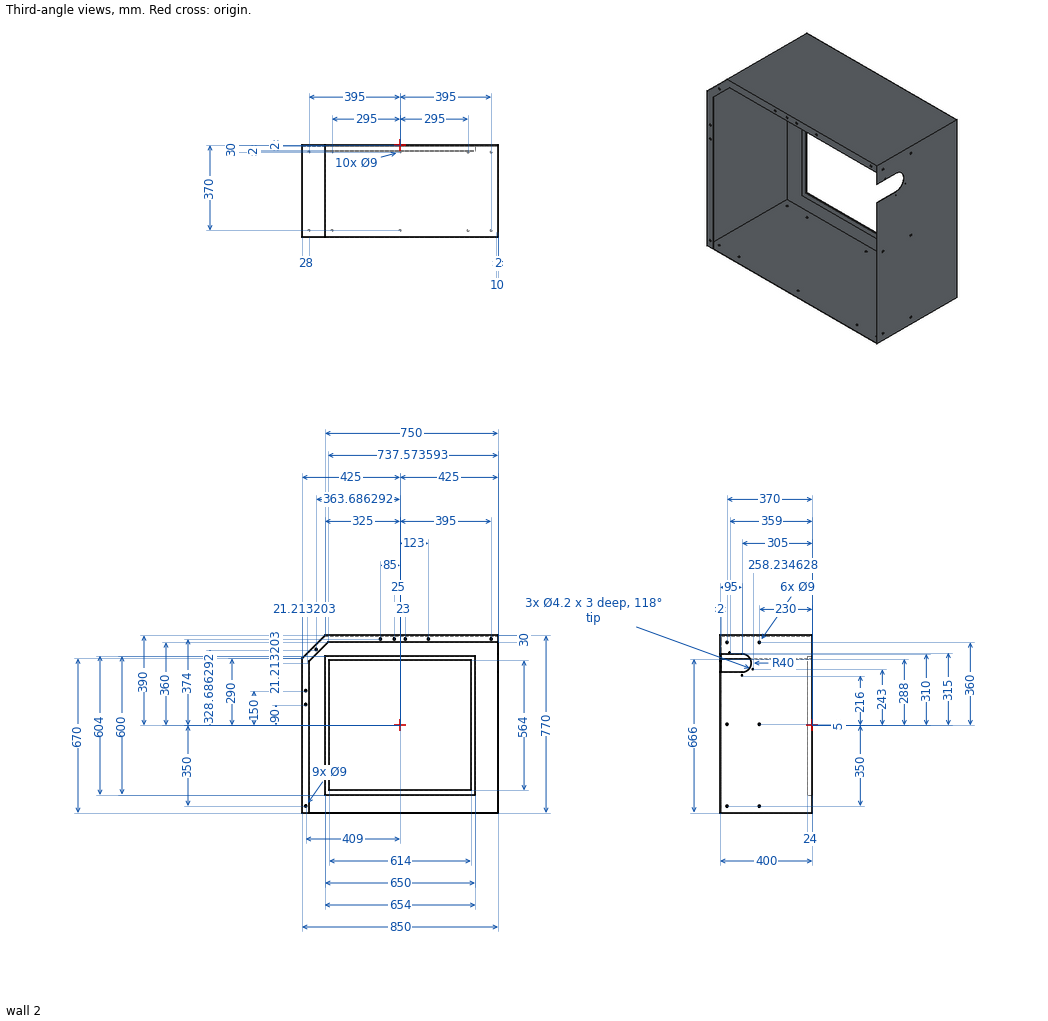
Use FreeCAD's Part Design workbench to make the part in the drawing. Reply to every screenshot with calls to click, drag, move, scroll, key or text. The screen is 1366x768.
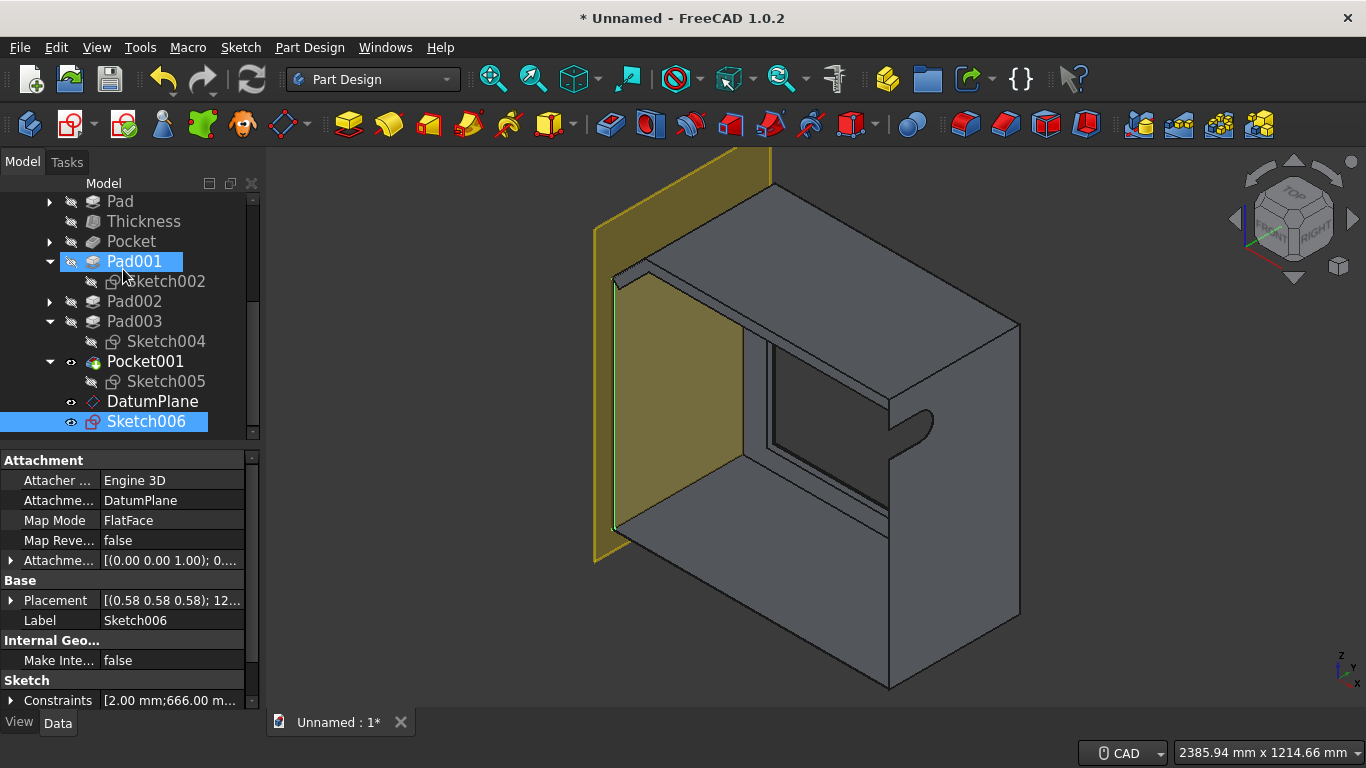
click(350, 124)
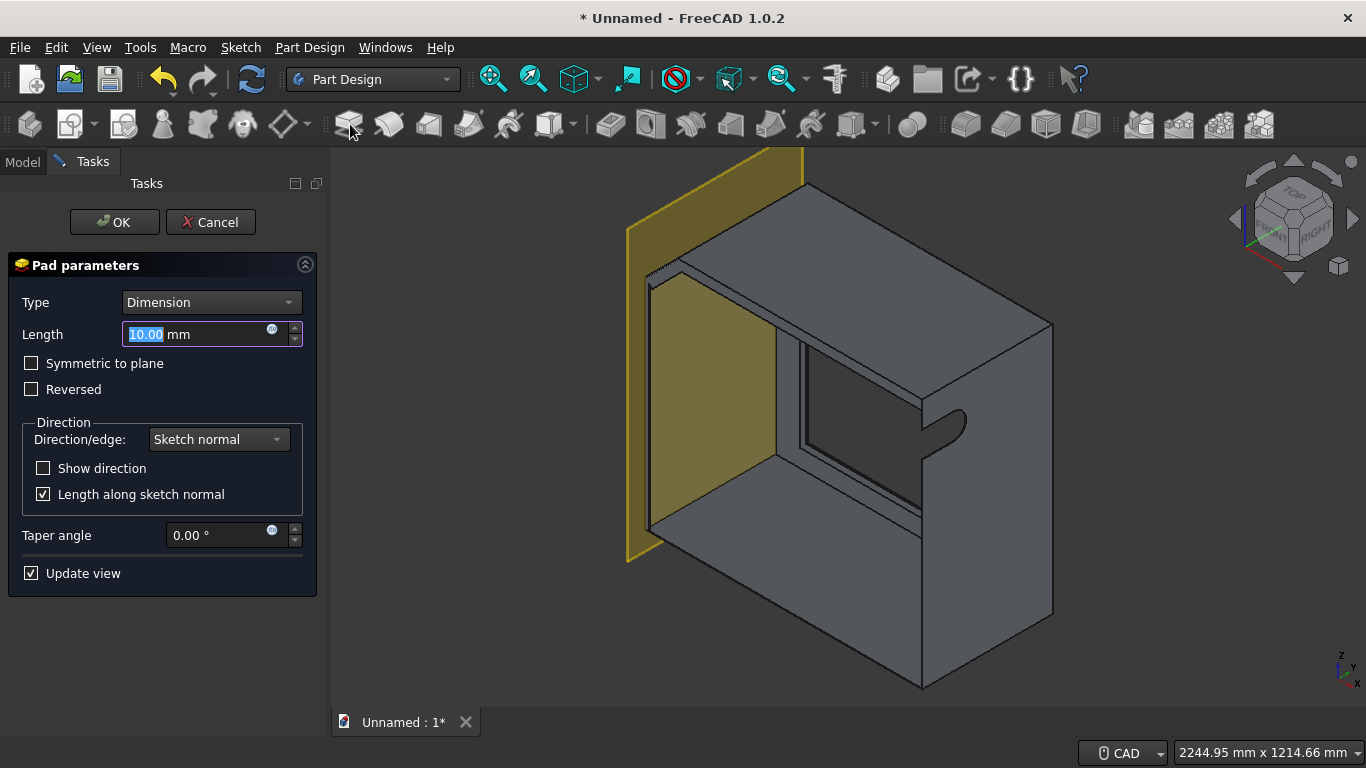
text(28)
key(Tab)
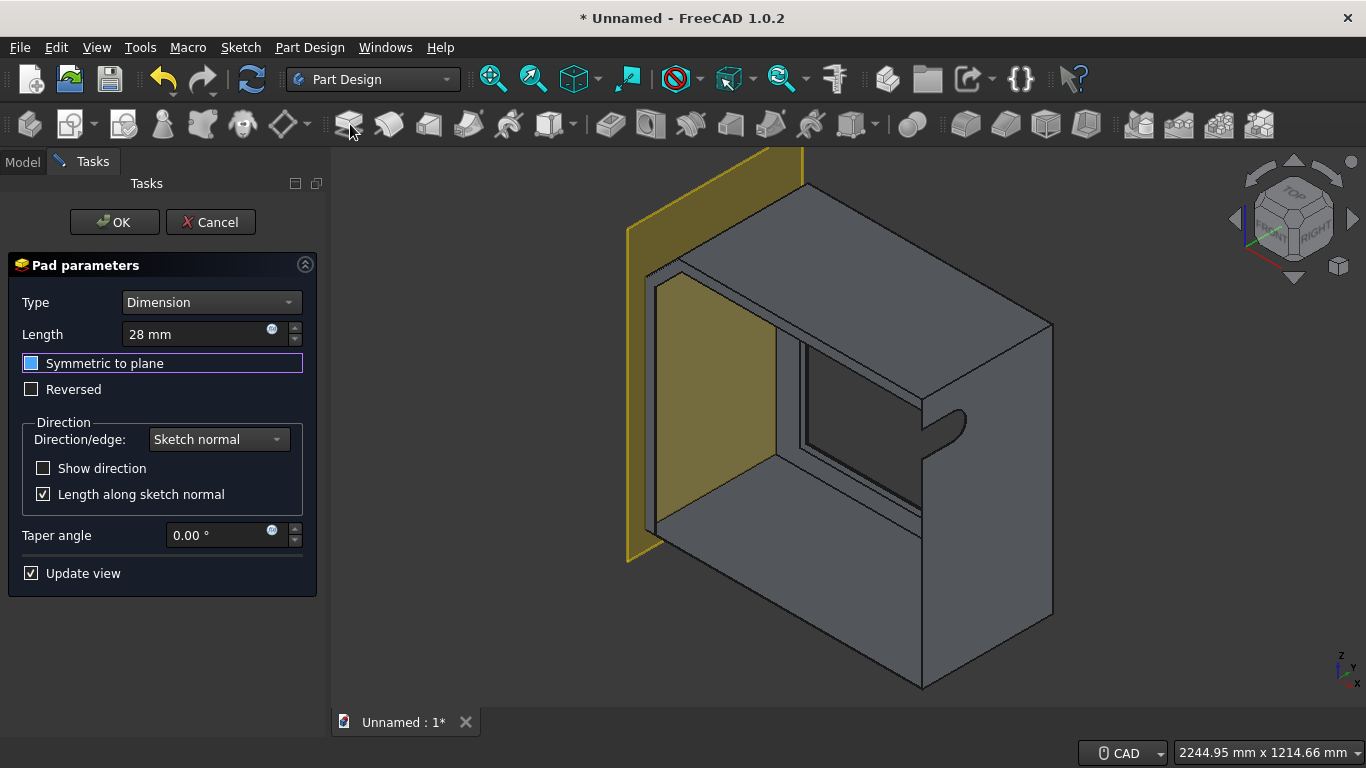
click(115, 222)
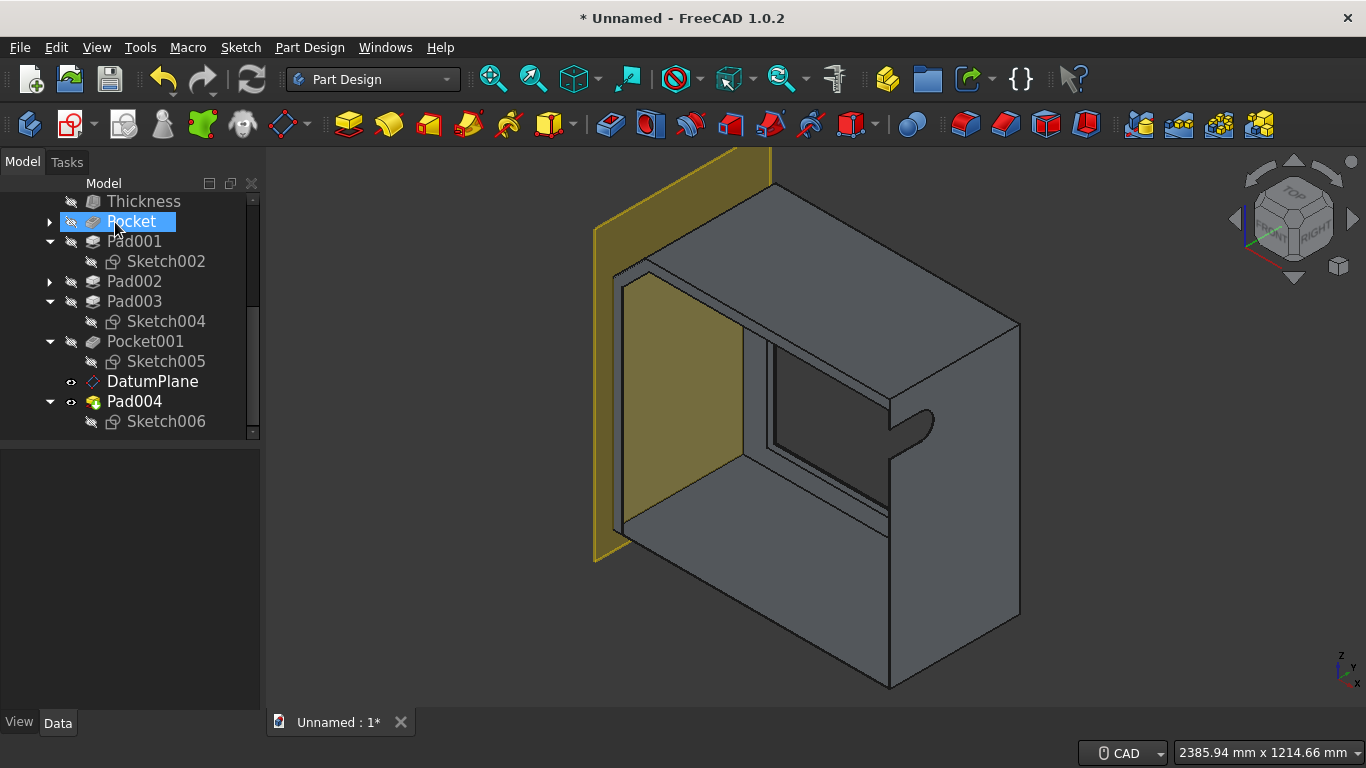
click(116, 382)
key(space)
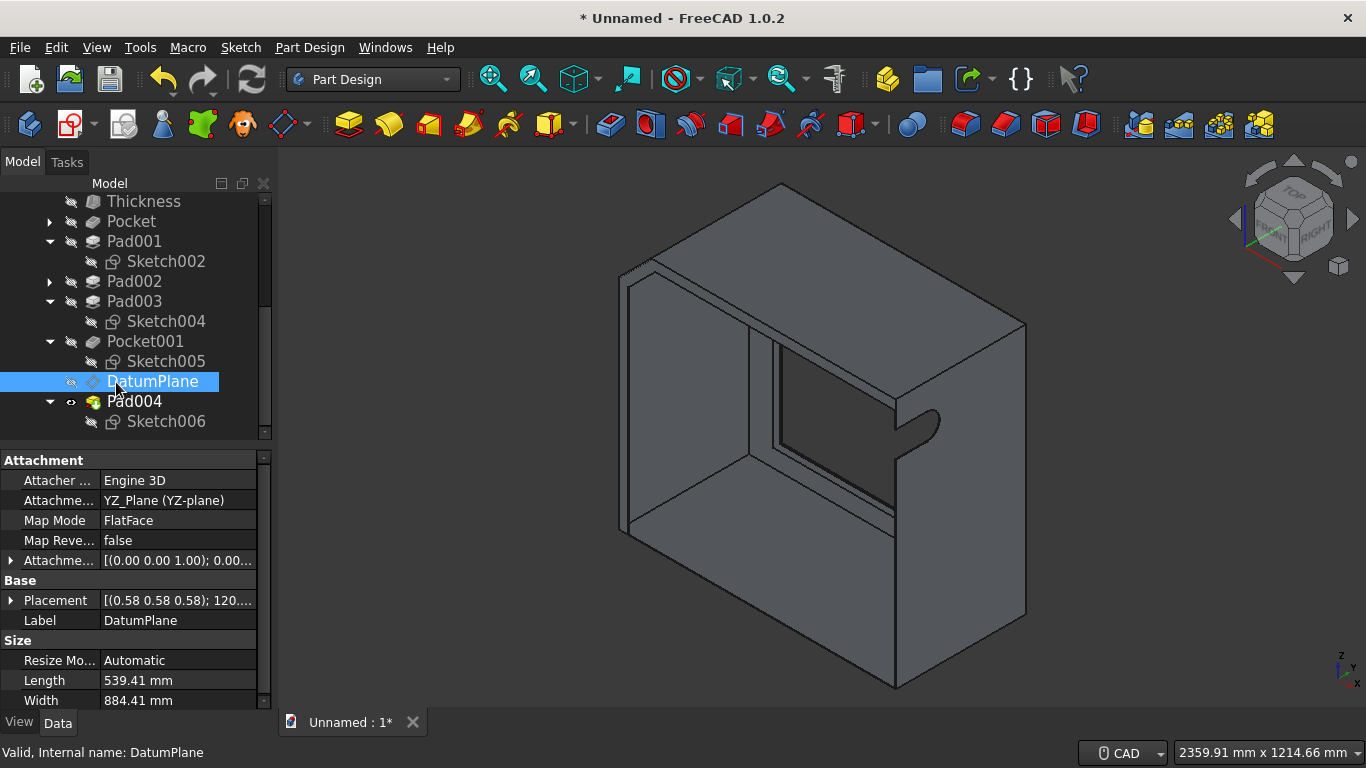
scroll(140, 317, down, 3)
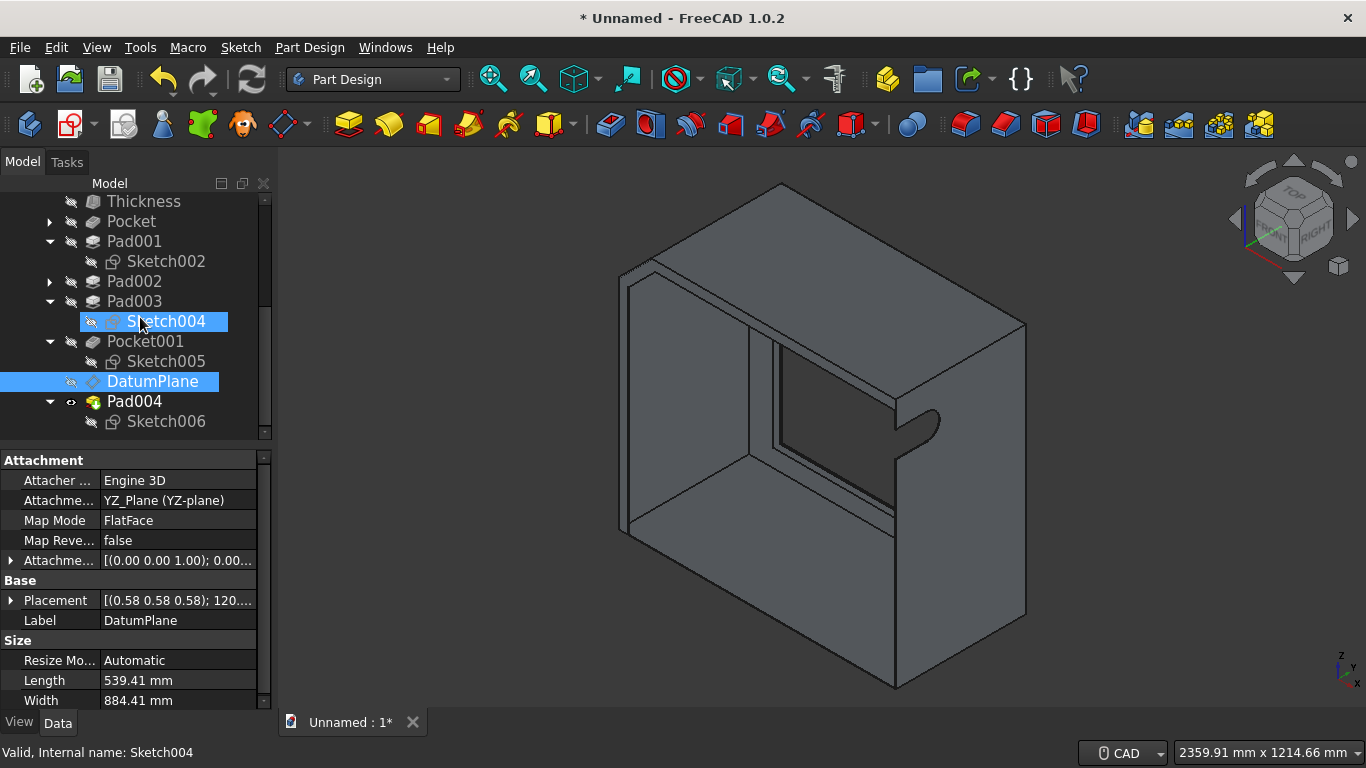
scroll(140, 317, up, 15)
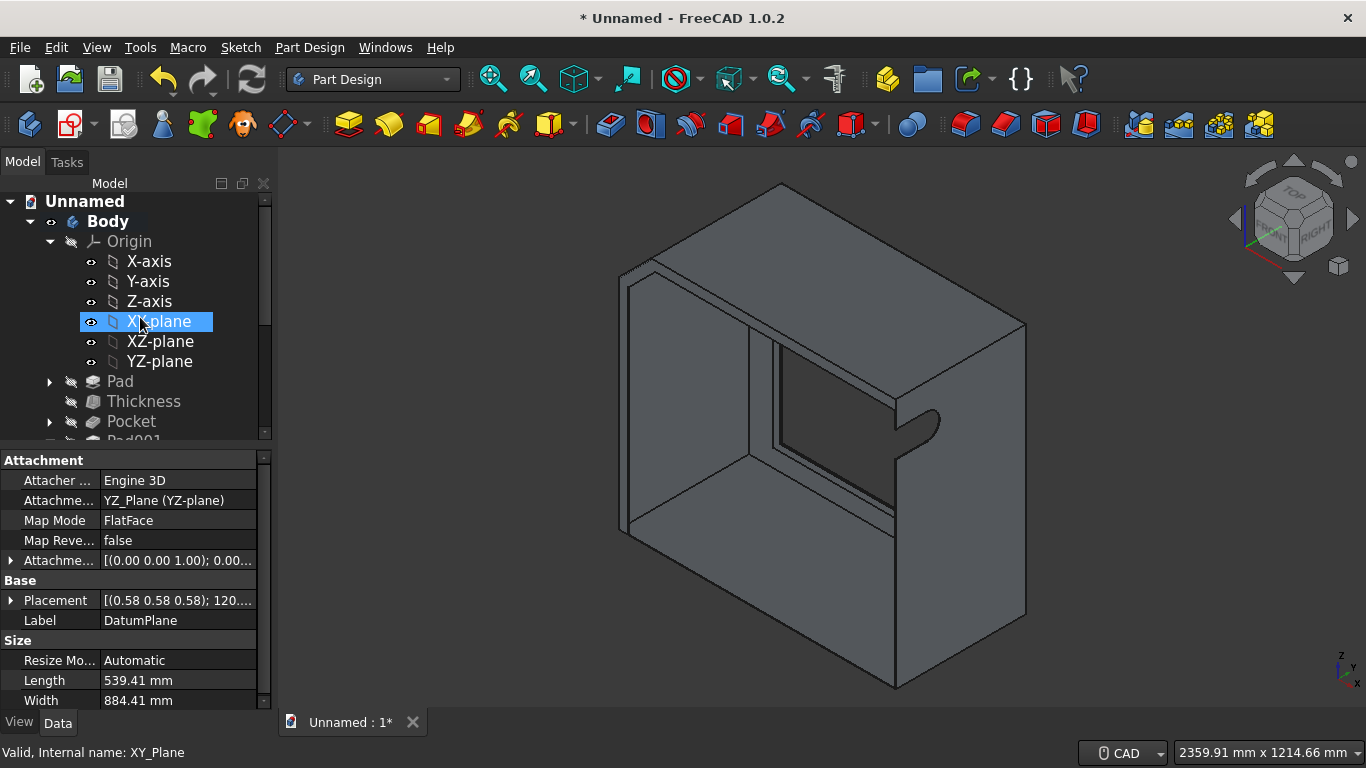
click(136, 342)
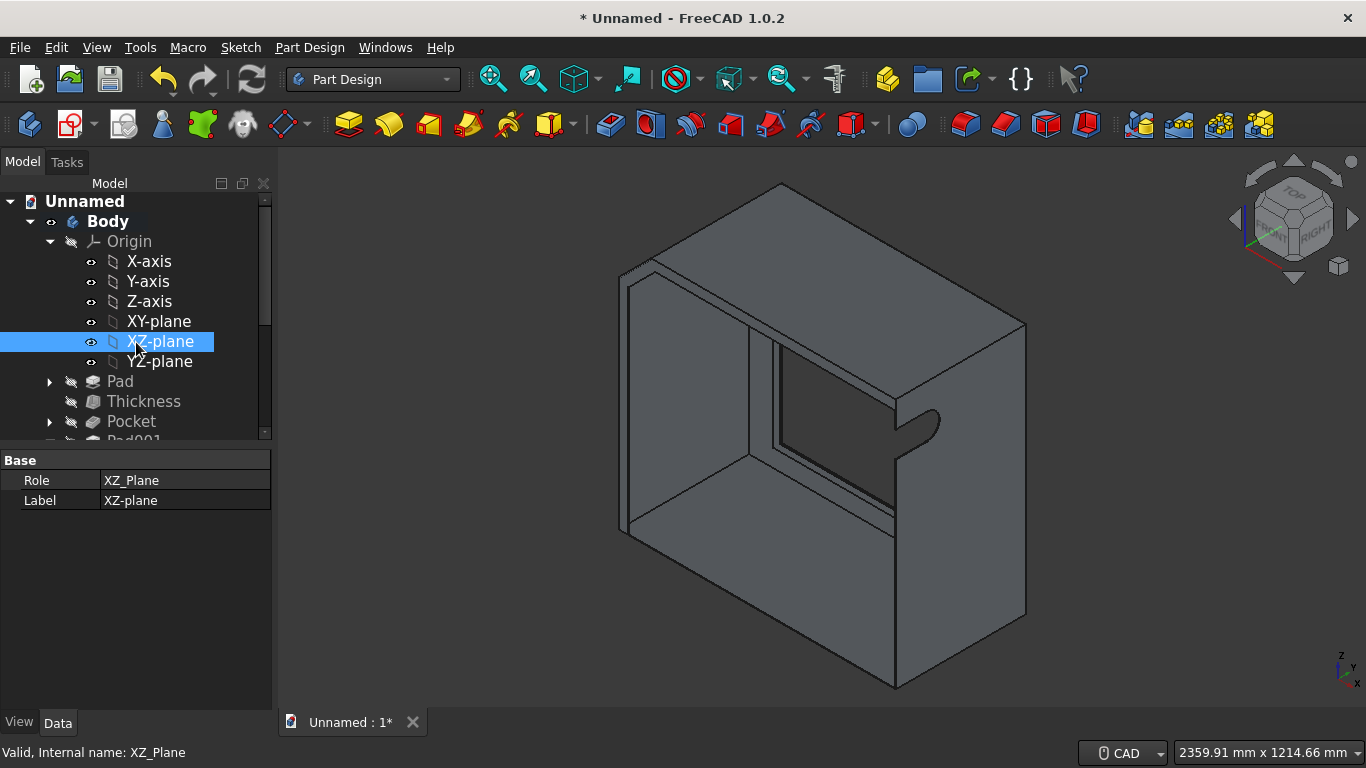
click(284, 124)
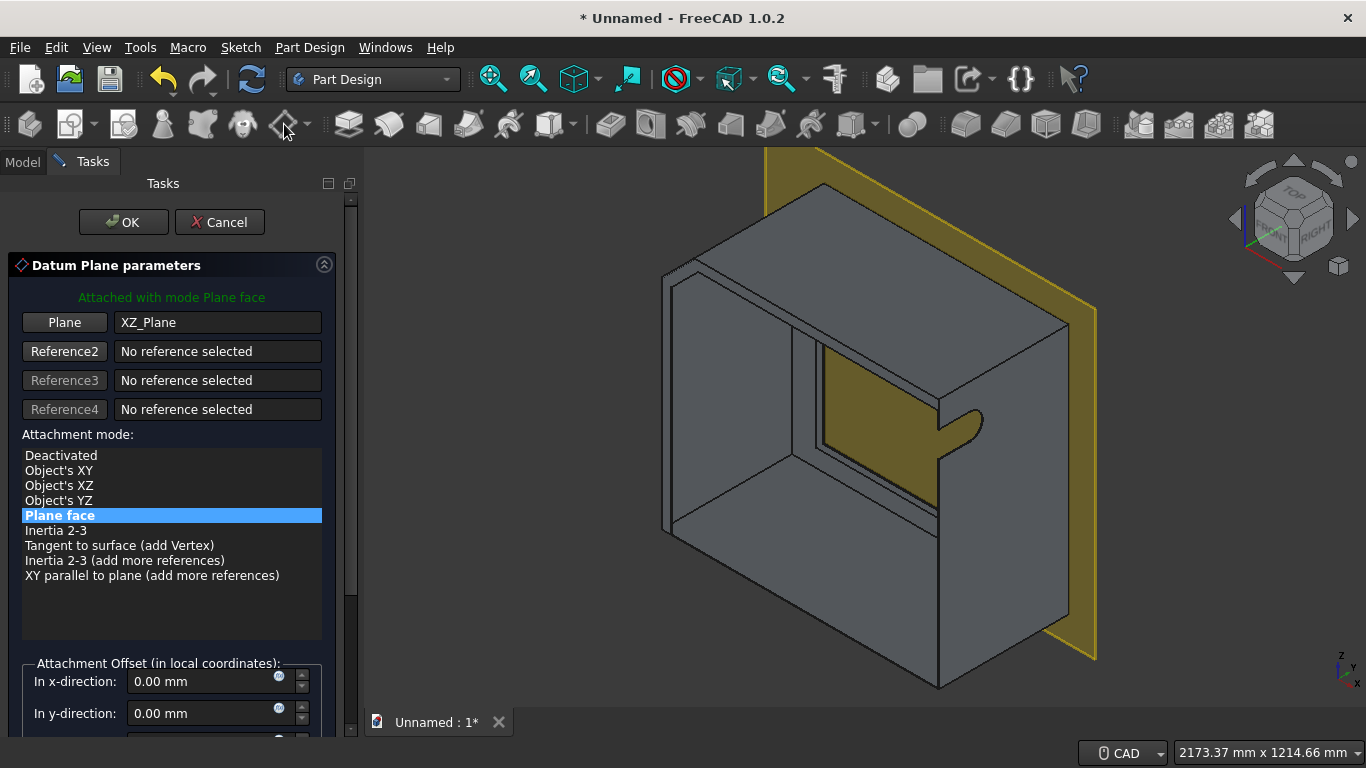
scroll(351, 464, down, 2)